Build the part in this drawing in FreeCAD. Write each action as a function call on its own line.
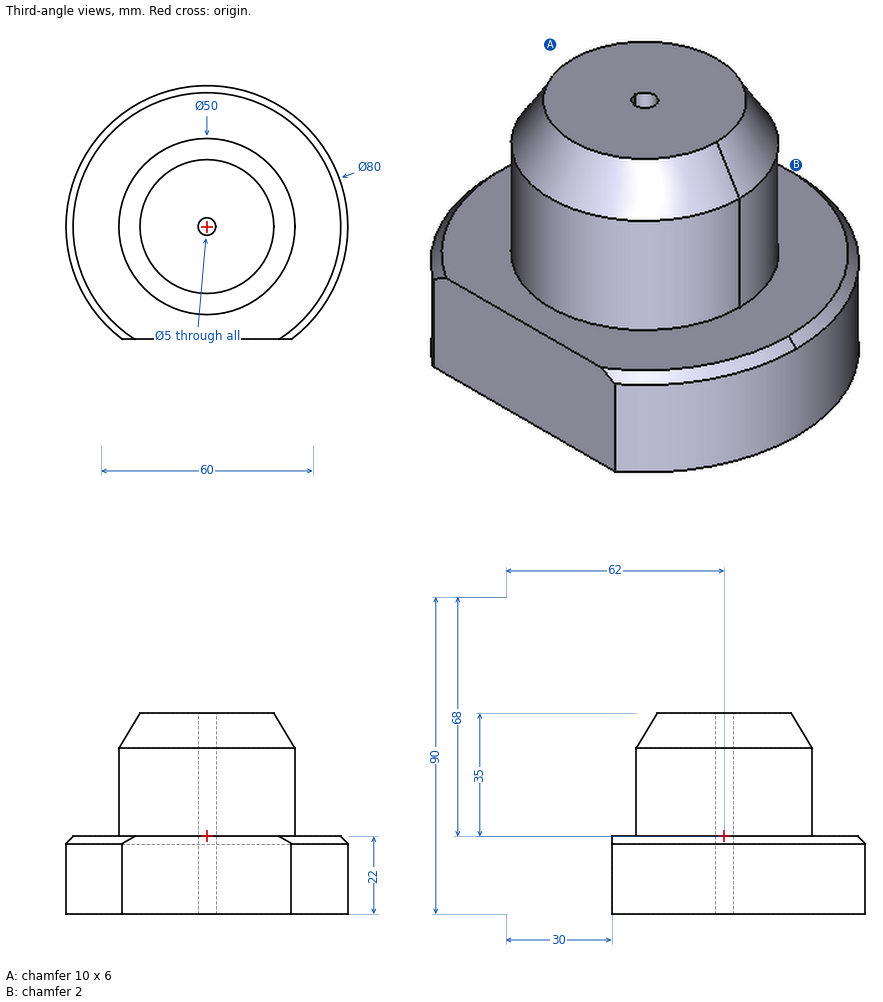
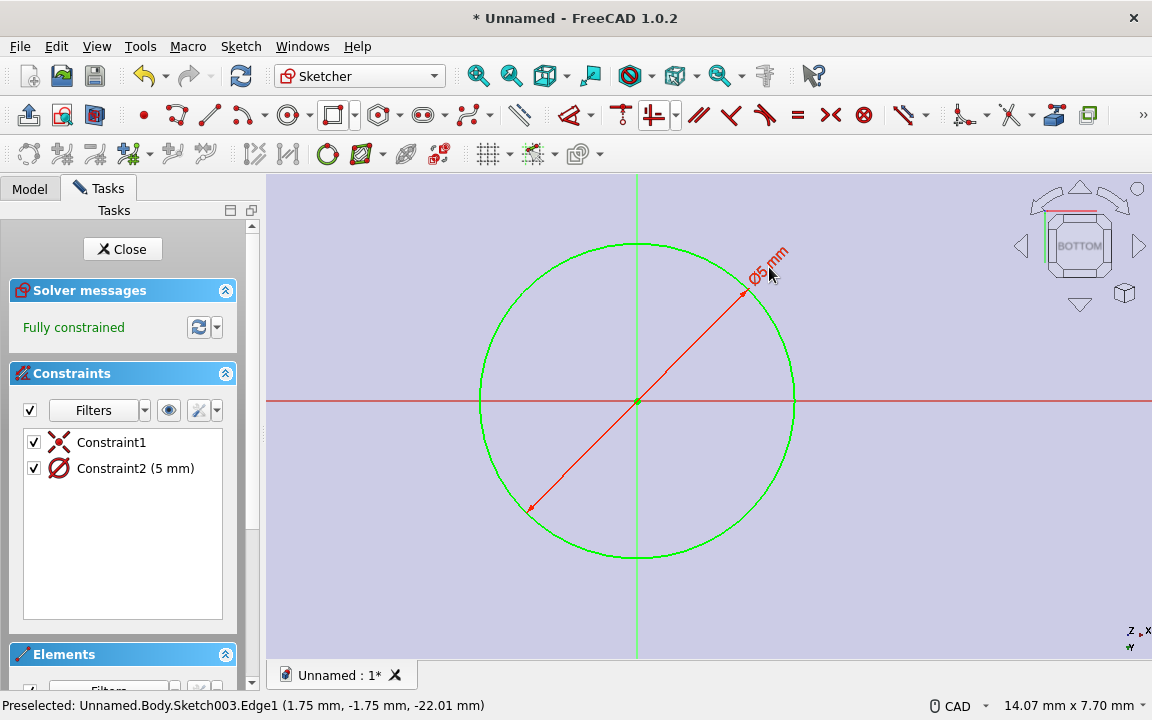
click(123, 249)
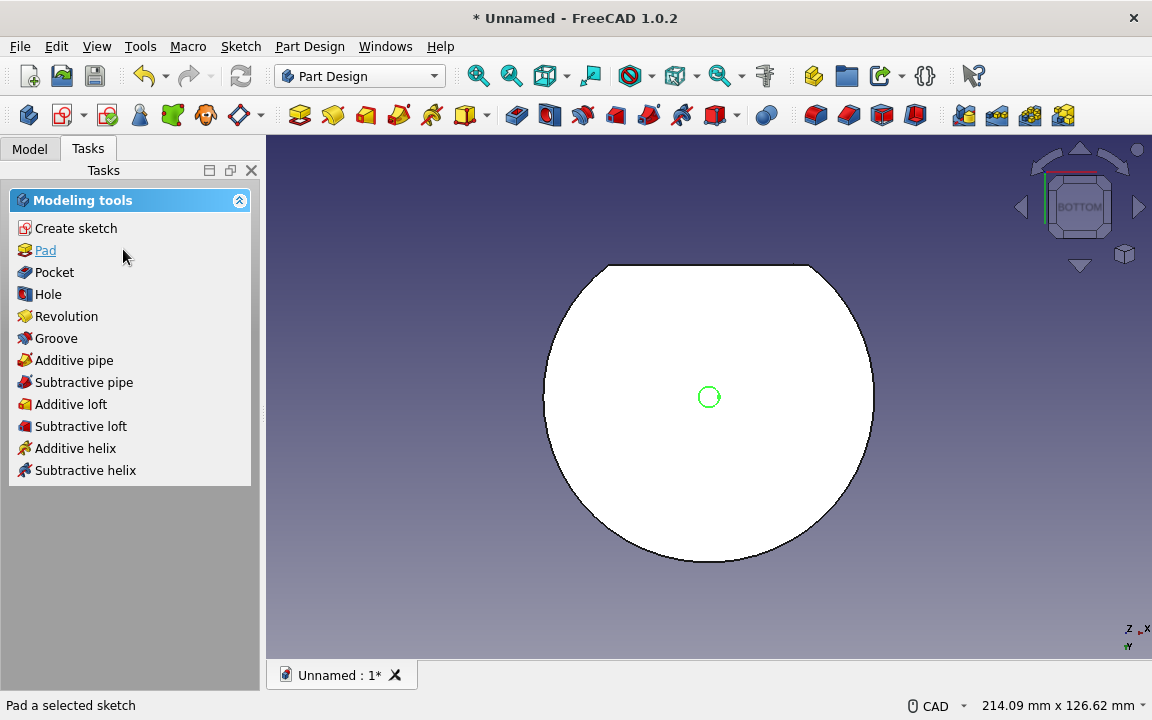
click(550, 116)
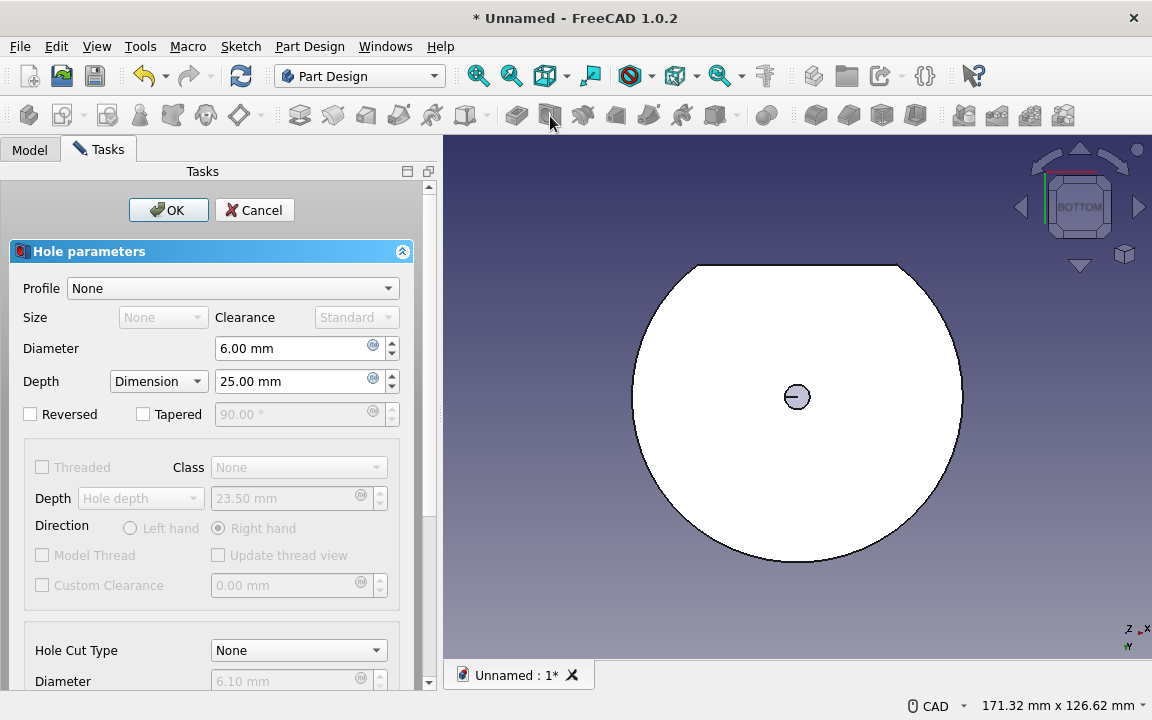
triple_click(300, 348)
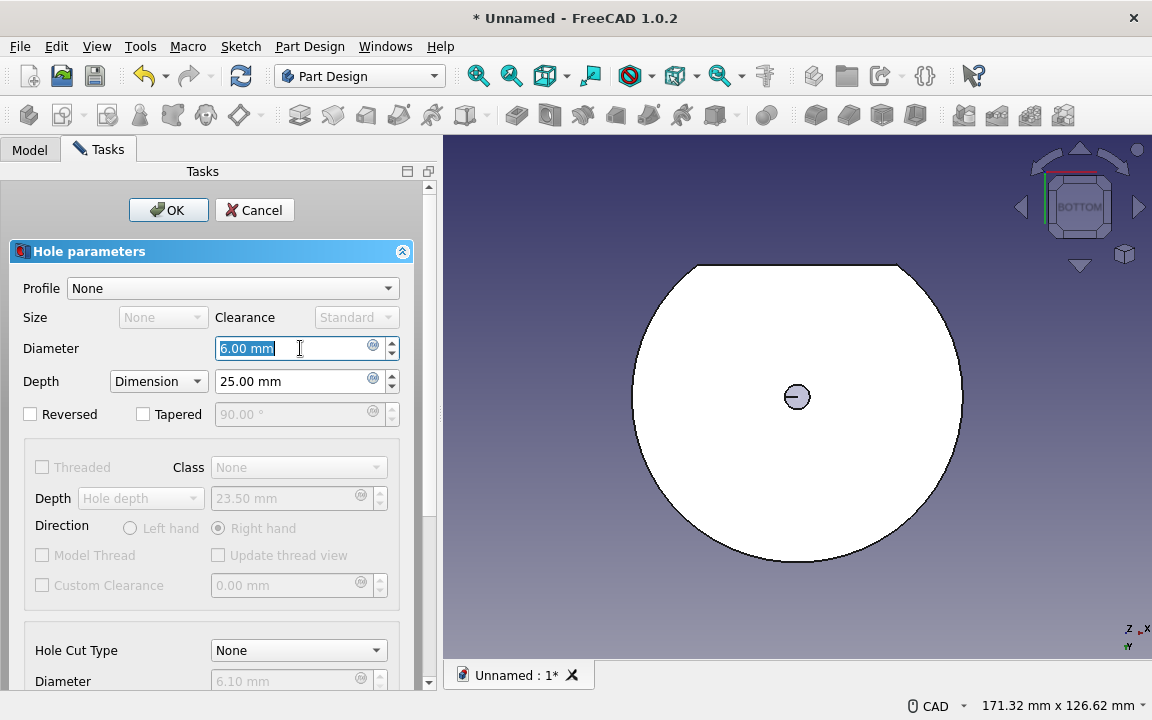
text(5)
key(Tab)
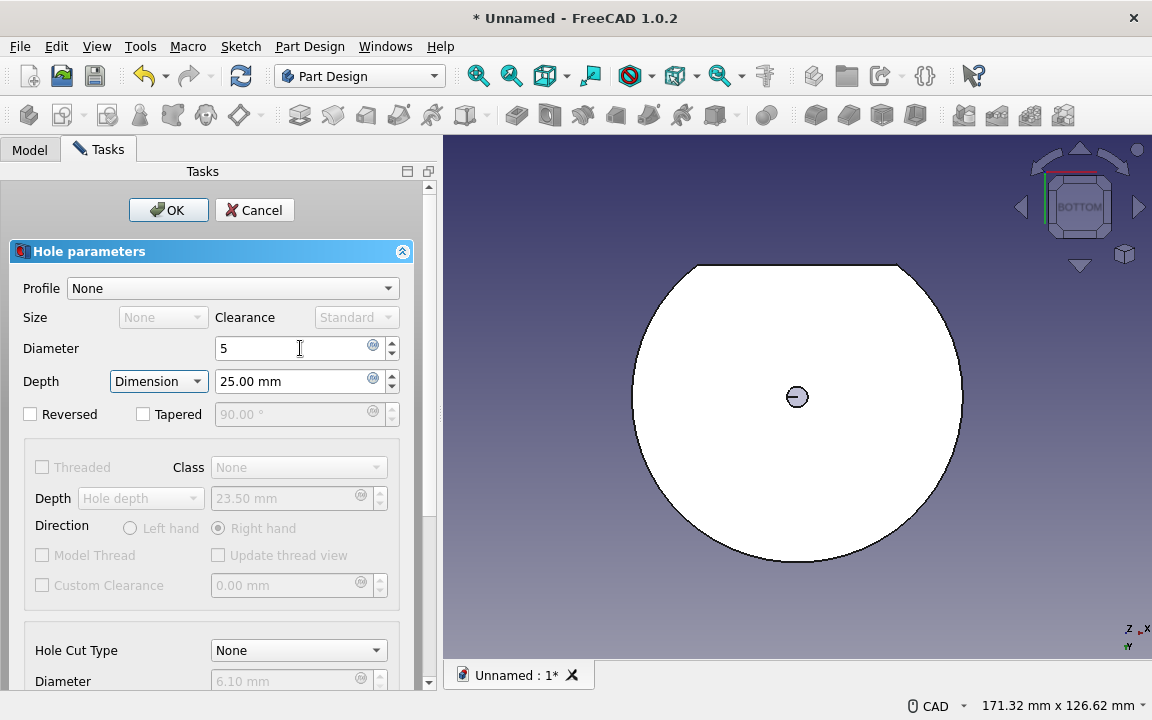
click(160, 382)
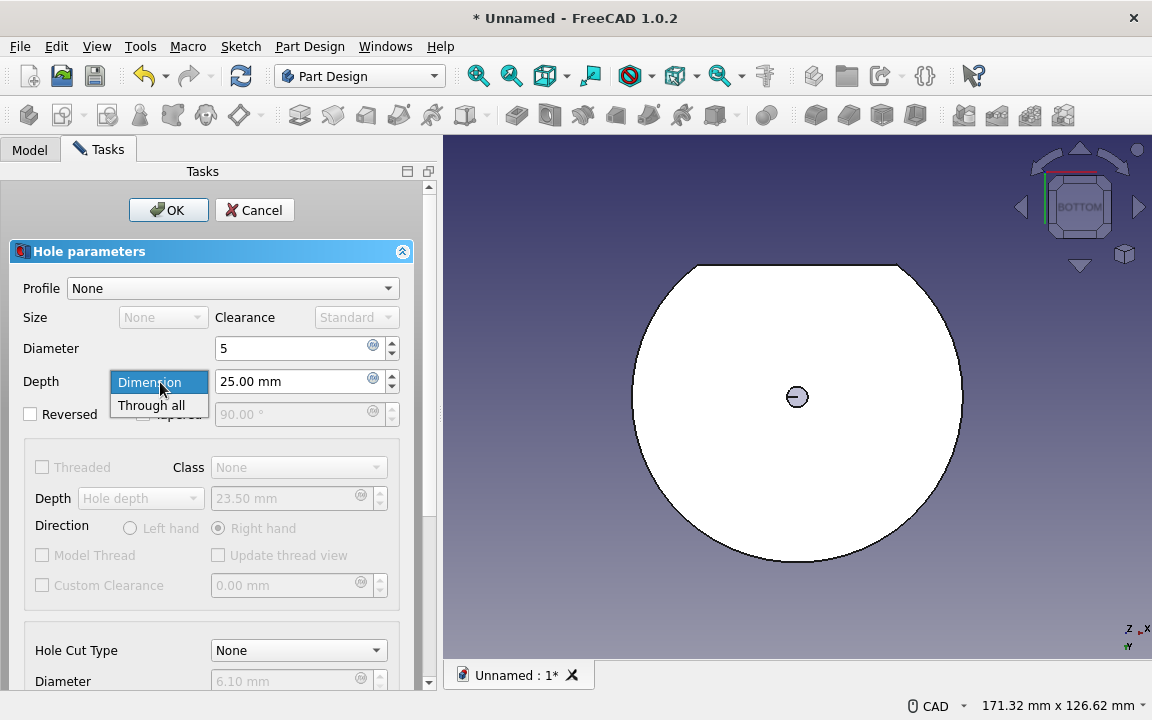
click(158, 406)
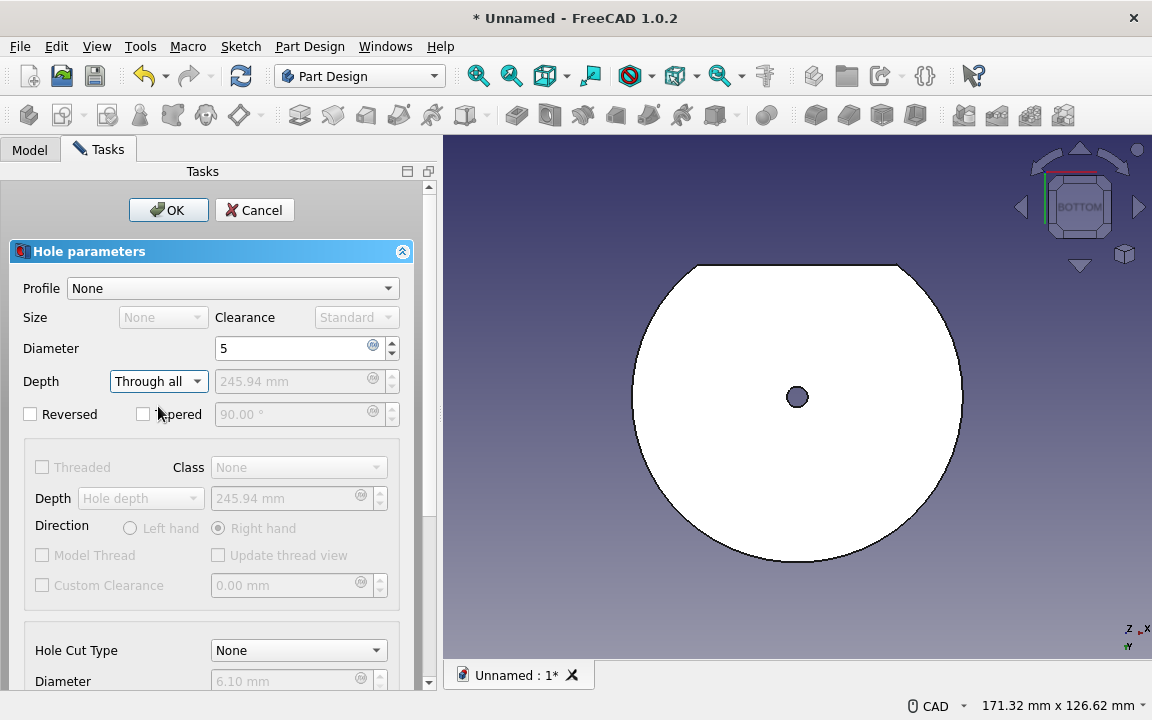
click(169, 210)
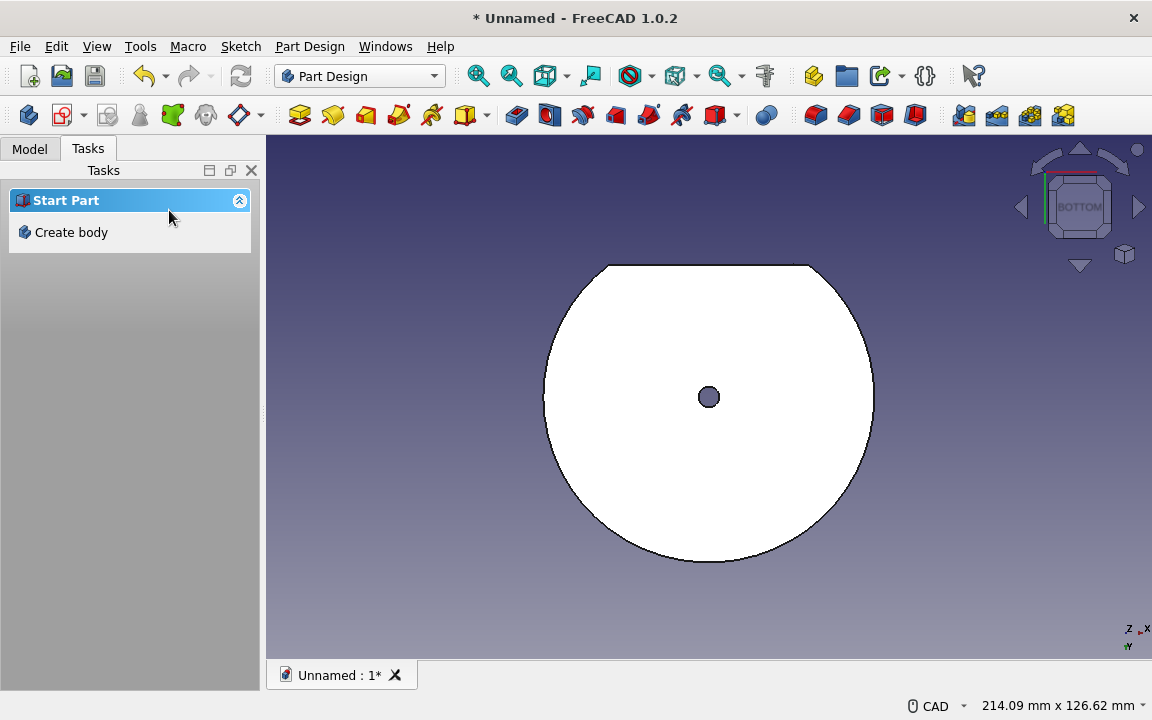
key(0)